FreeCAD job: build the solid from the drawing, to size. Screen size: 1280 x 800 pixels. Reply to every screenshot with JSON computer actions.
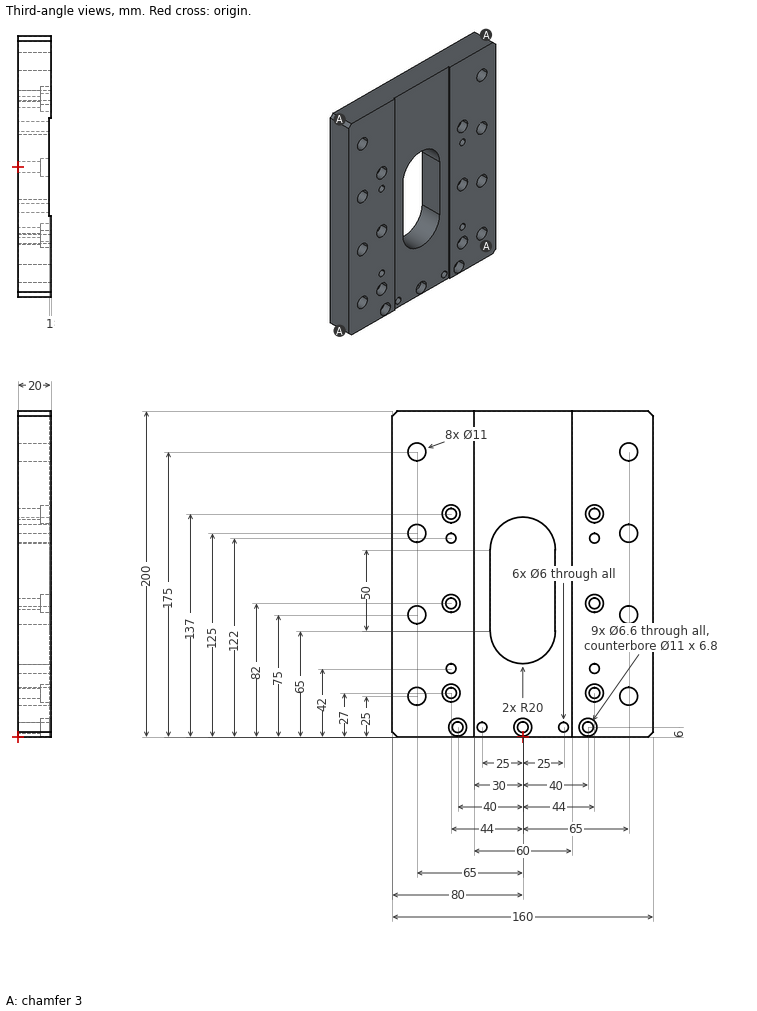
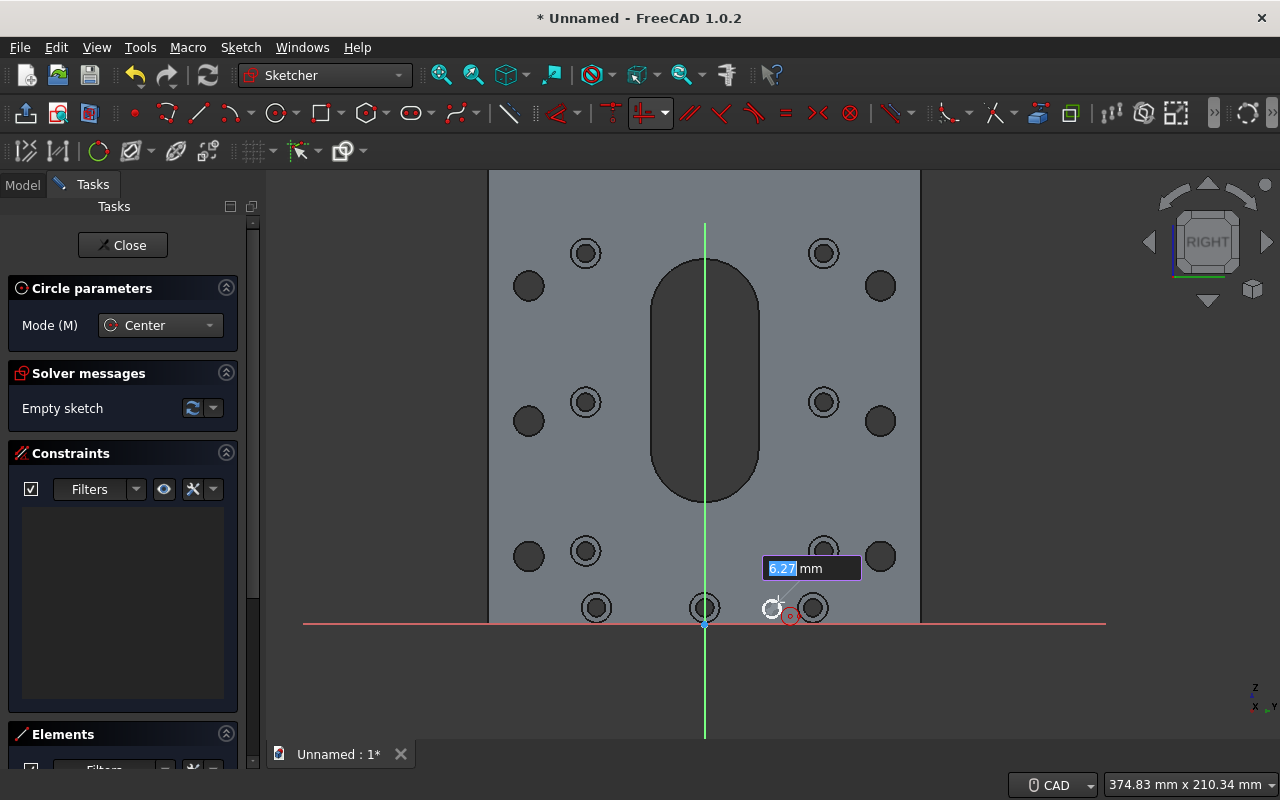
{"action": "type", "text": "6"}
{"action": "key", "text": "Return"}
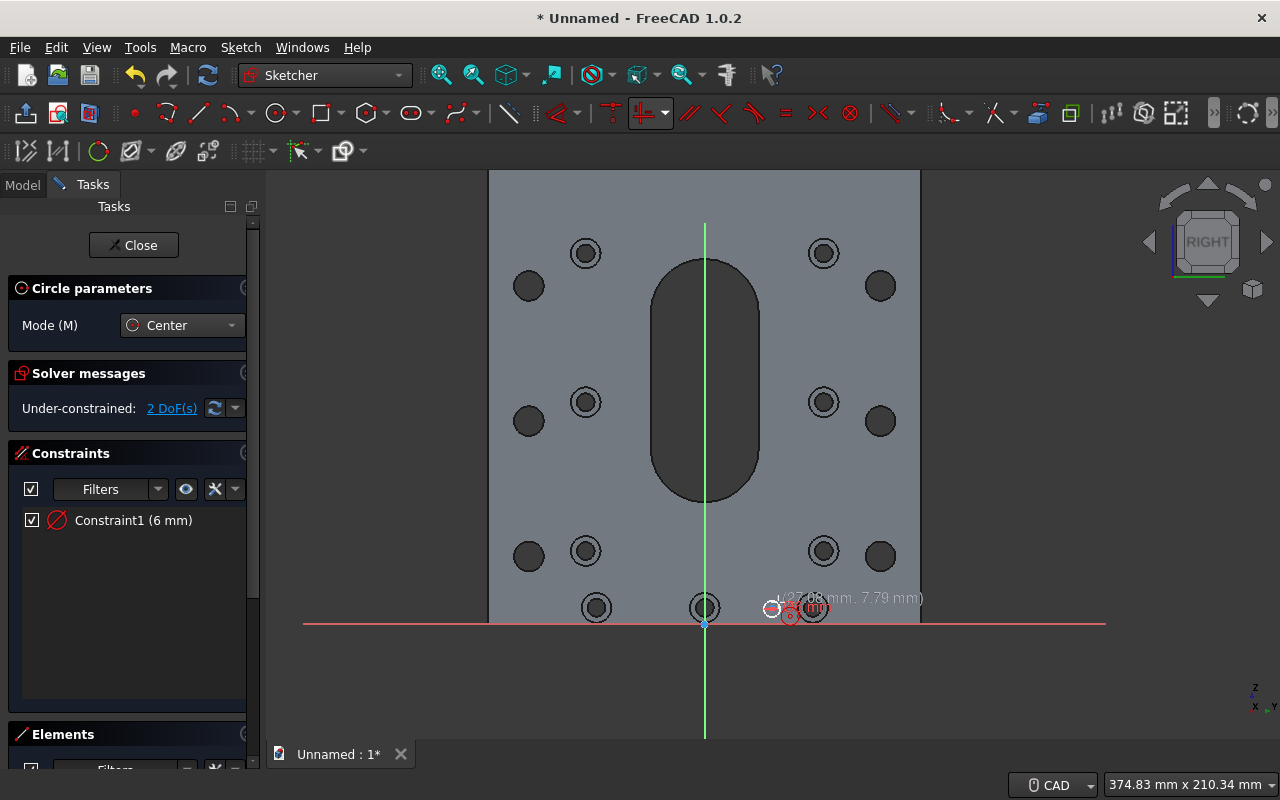
{"action": "scroll", "coordinate": [637, 608], "scroll_direction": "up", "scroll_amount": 6}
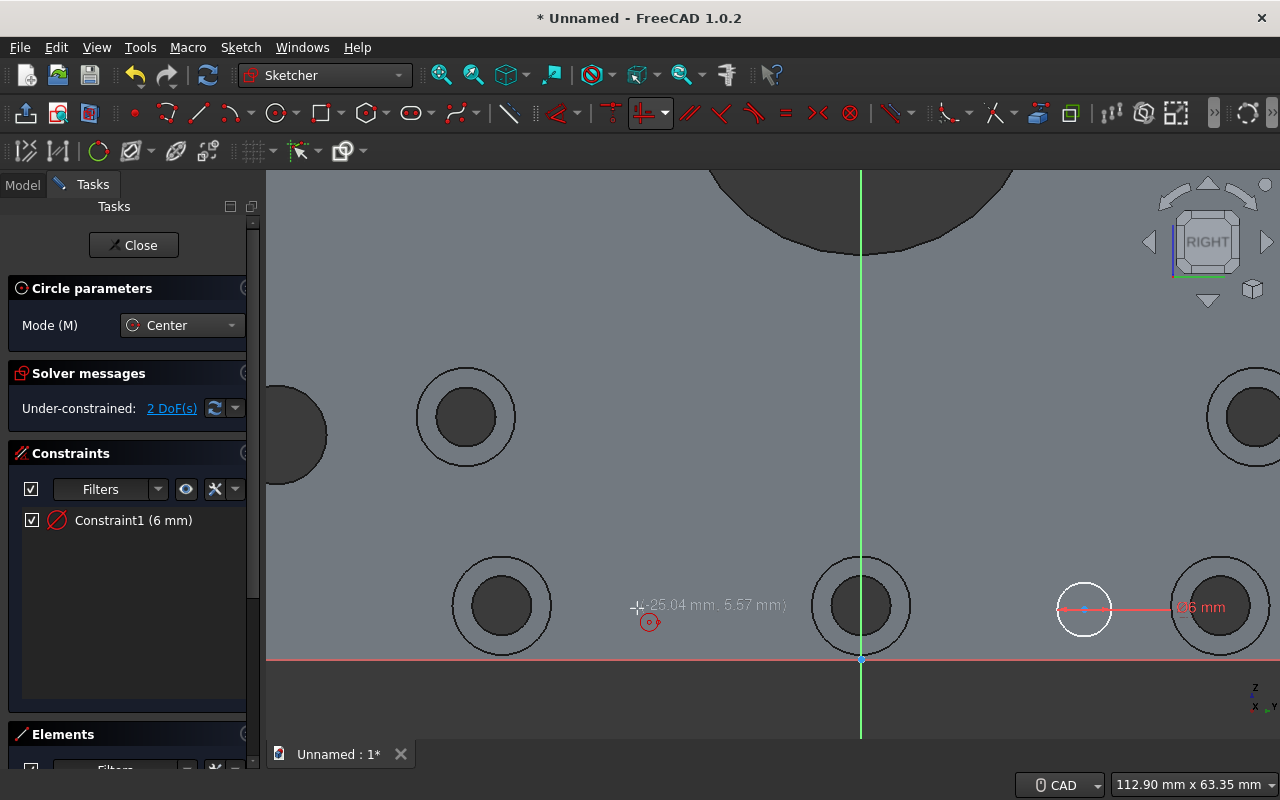
{"action": "scroll", "coordinate": [637, 608], "scroll_direction": "down", "scroll_amount": 6}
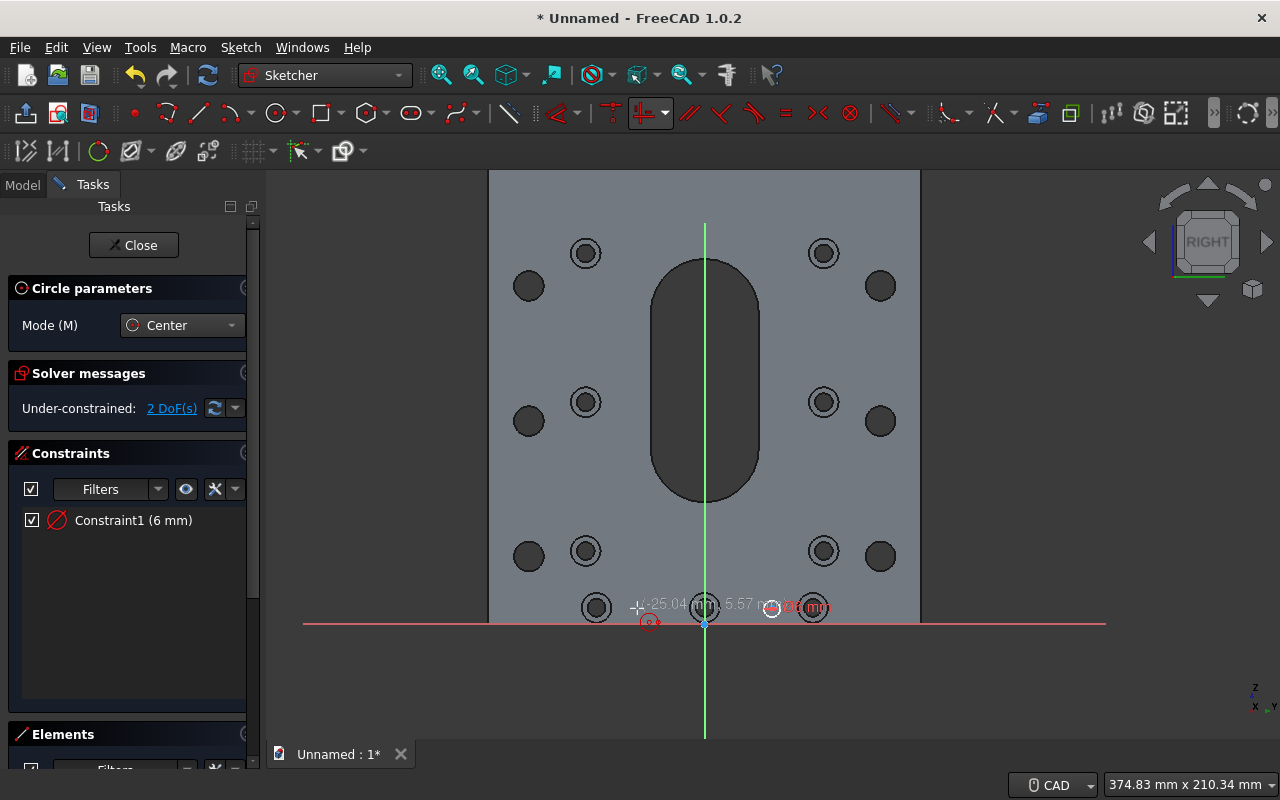
{"action": "left_click", "coordinate": [637, 608]}
{"action": "mouse_move", "coordinate": [643, 602]}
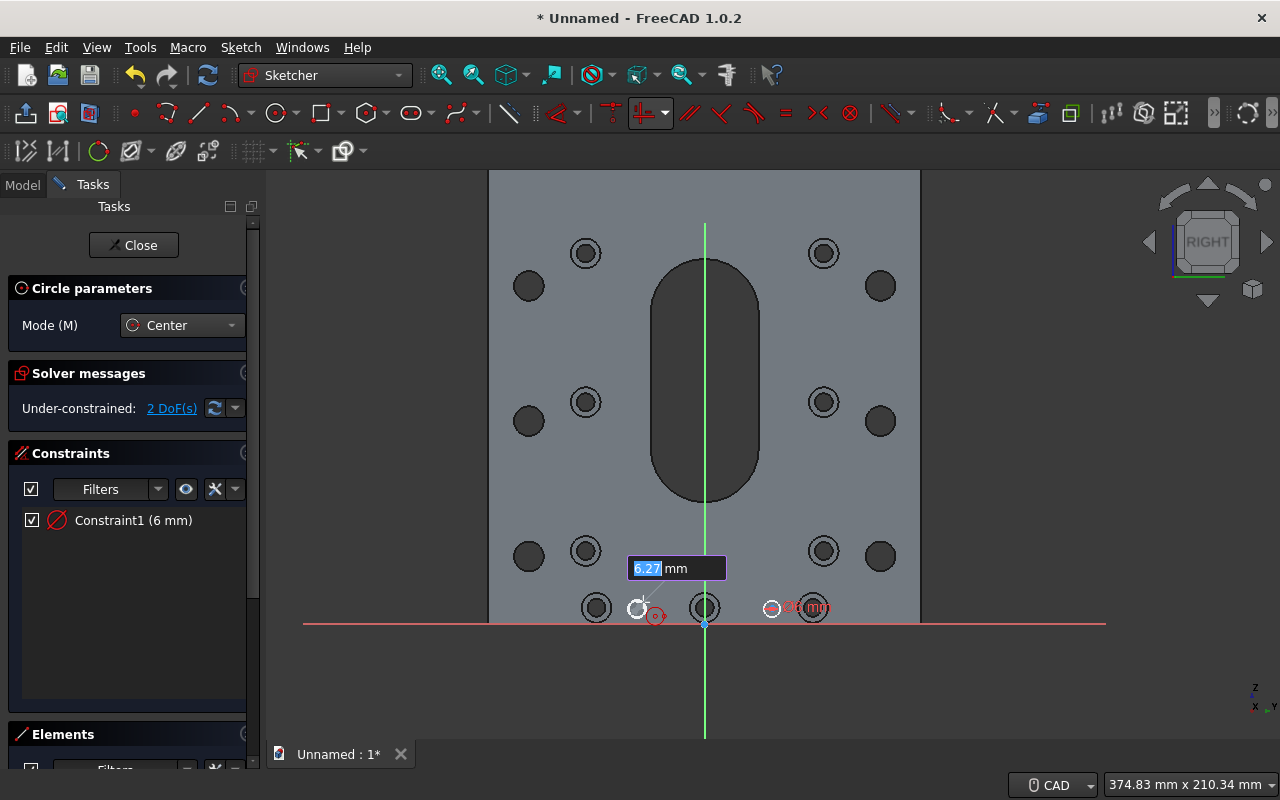
{"action": "type", "text": "6"}
{"action": "key", "text": "Return"}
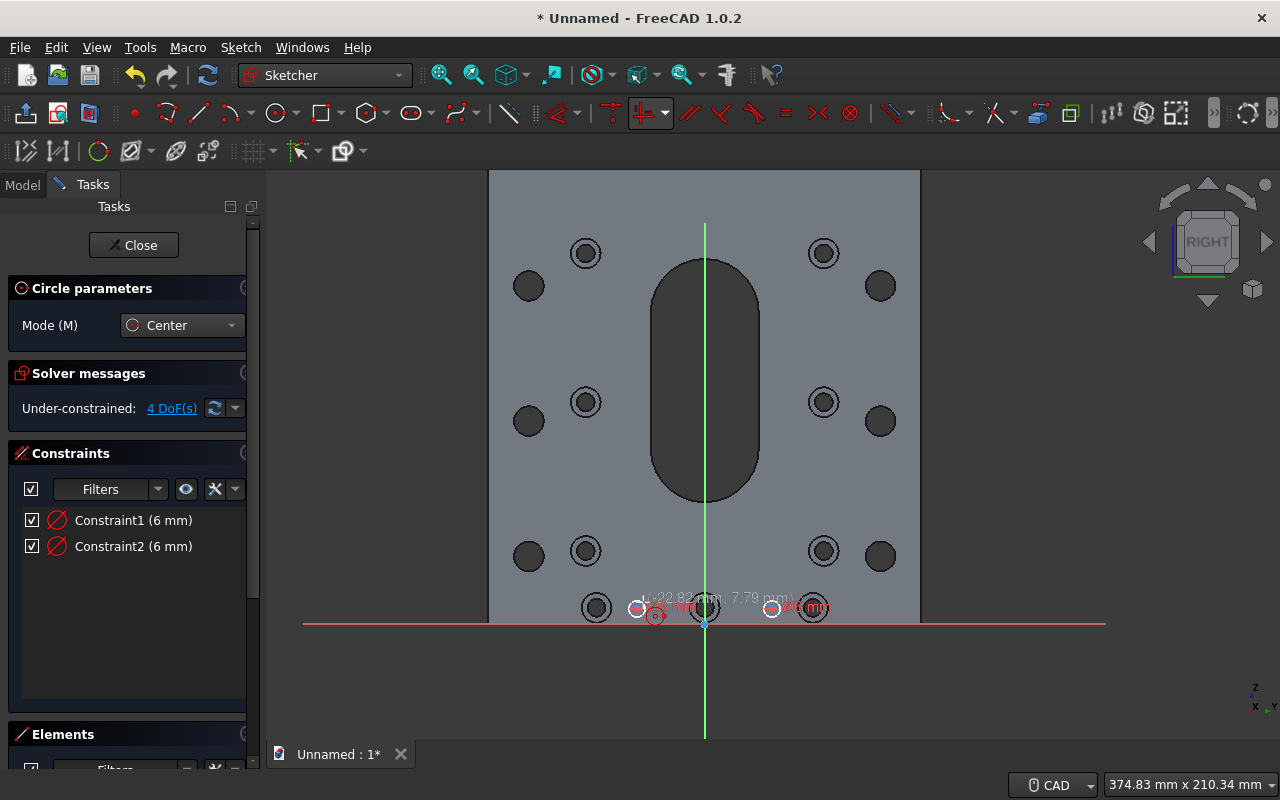
{"action": "scroll", "coordinate": [586, 510], "scroll_direction": "up", "scroll_amount": 6}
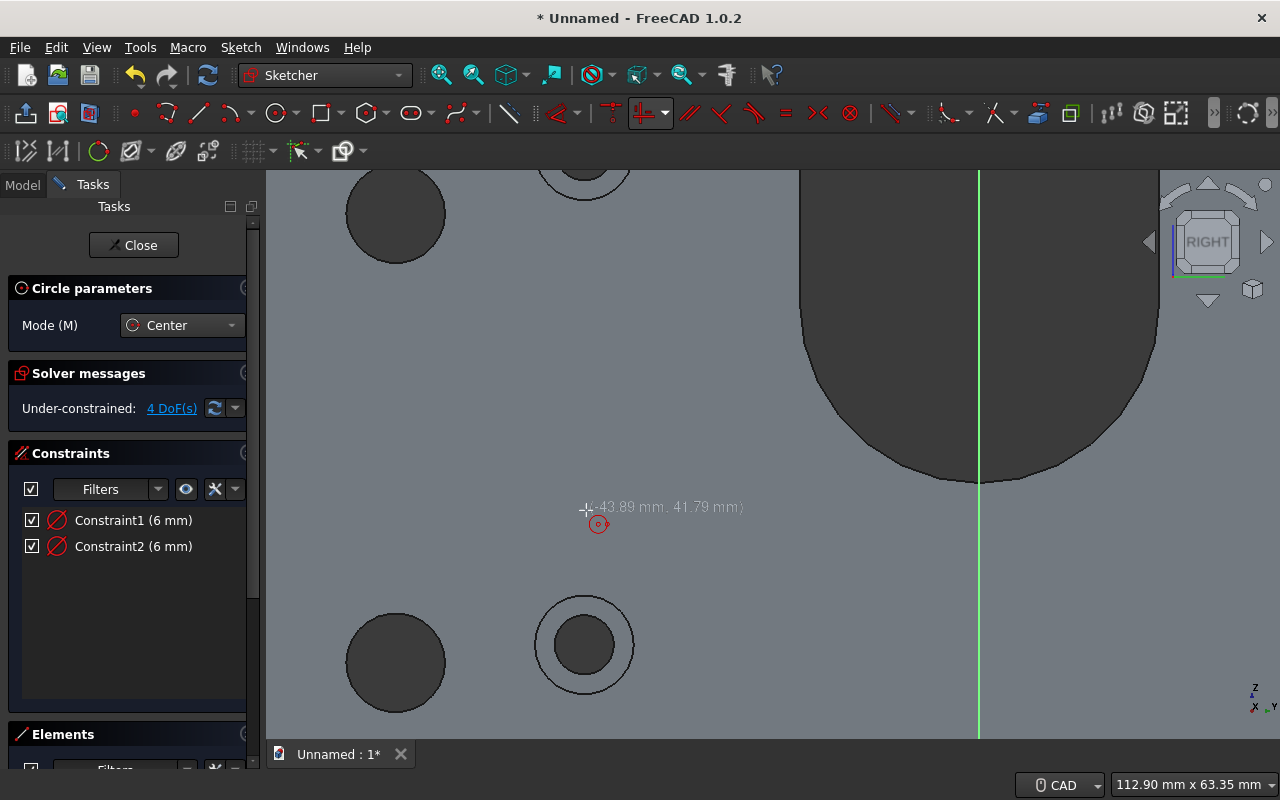
{"action": "scroll", "coordinate": [586, 510], "scroll_direction": "down", "scroll_amount": 6}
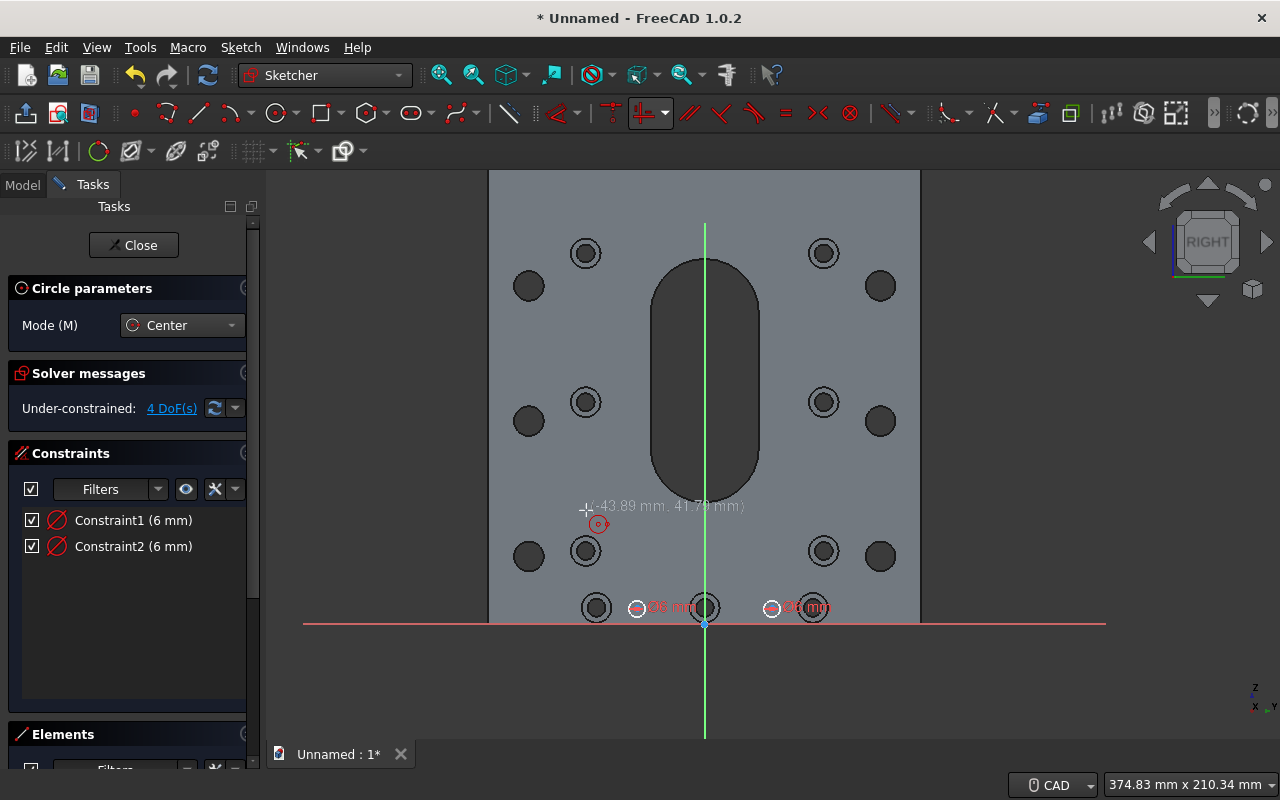
{"action": "left_click", "coordinate": [586, 510]}
{"action": "mouse_move", "coordinate": [591, 505]}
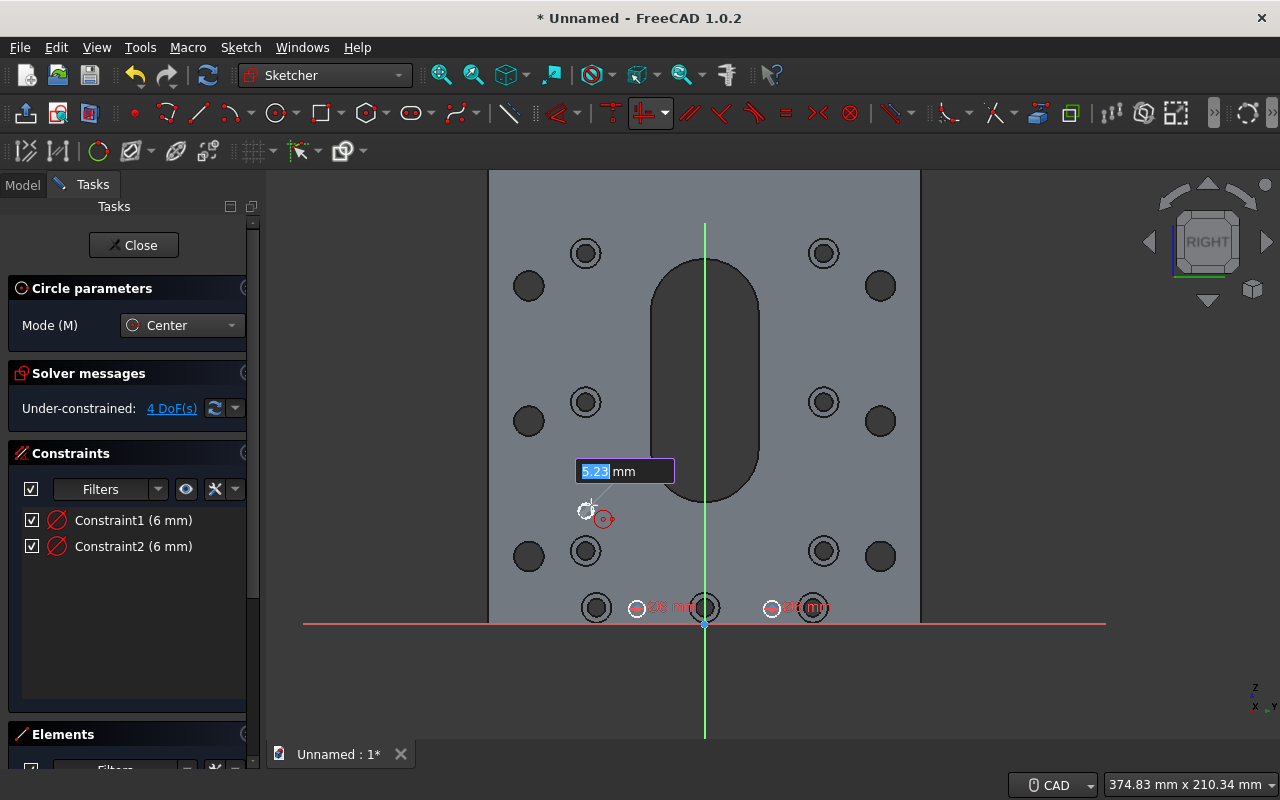
{"action": "type", "text": "6"}
{"action": "key", "text": "Return"}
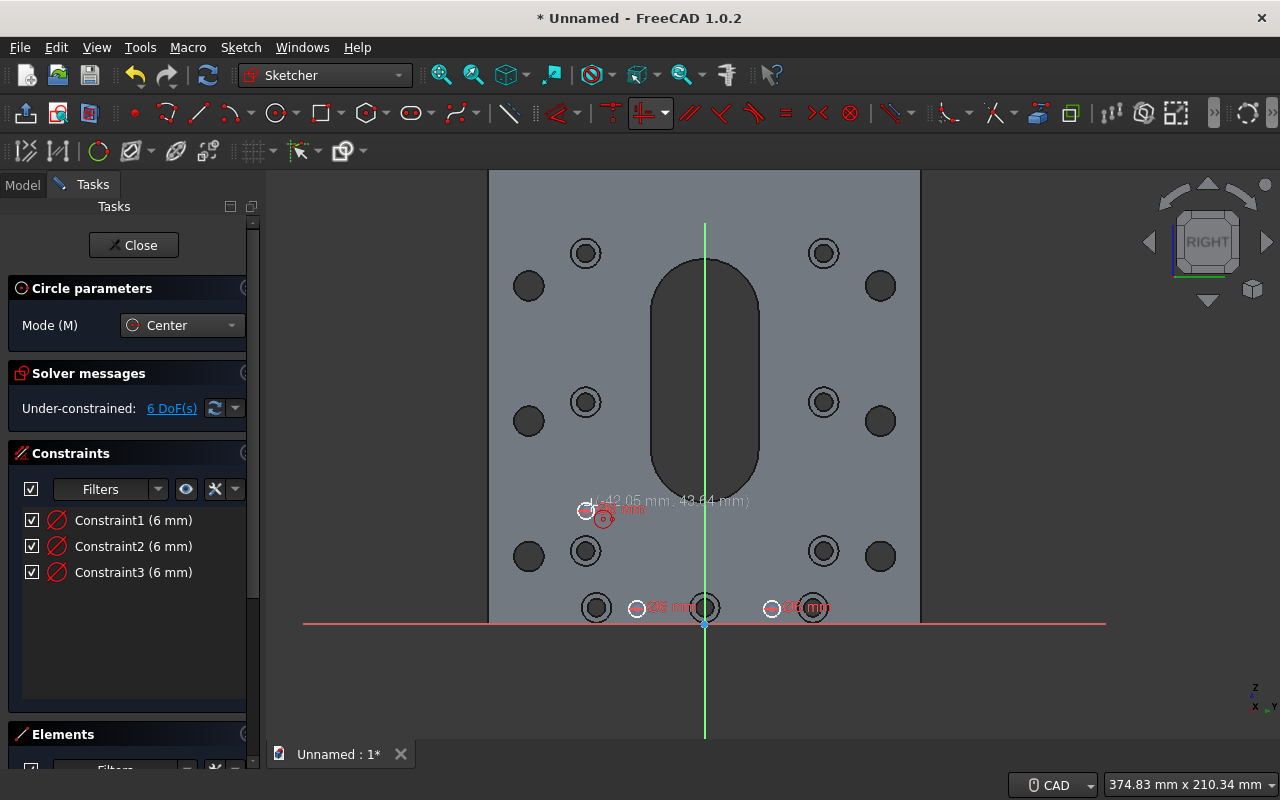
{"action": "scroll", "coordinate": [586, 294], "scroll_direction": "up", "scroll_amount": 6}